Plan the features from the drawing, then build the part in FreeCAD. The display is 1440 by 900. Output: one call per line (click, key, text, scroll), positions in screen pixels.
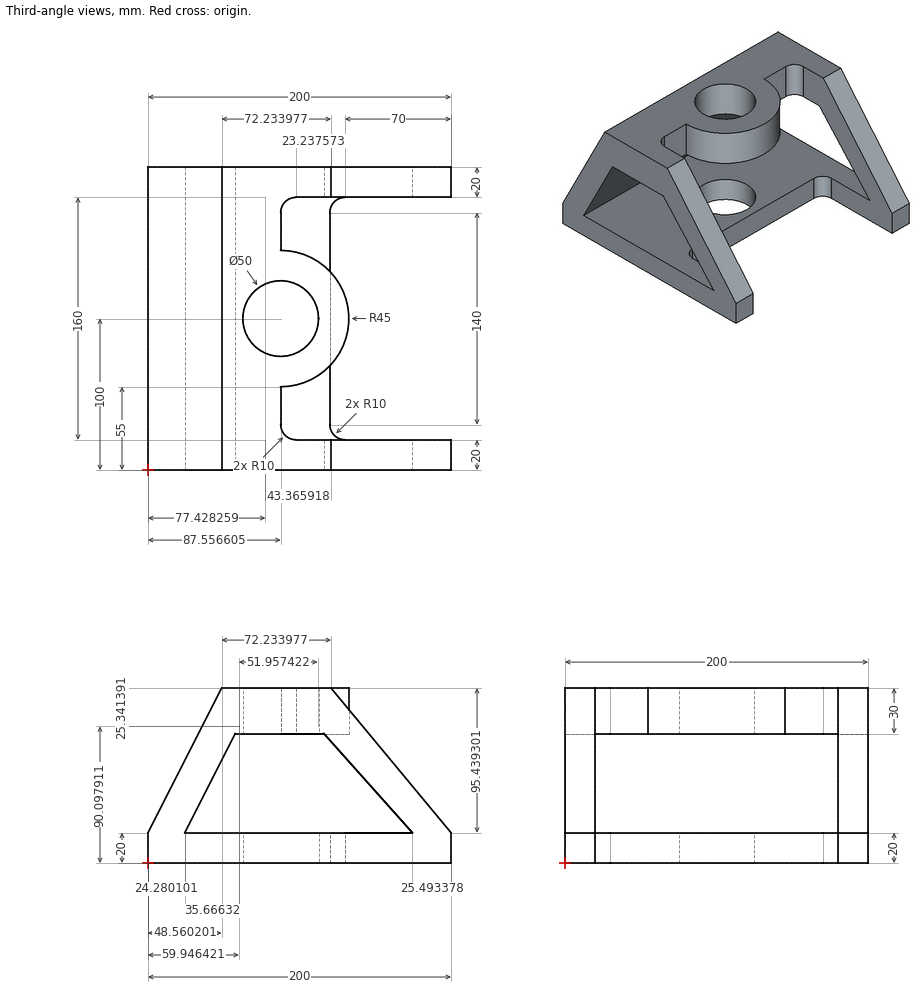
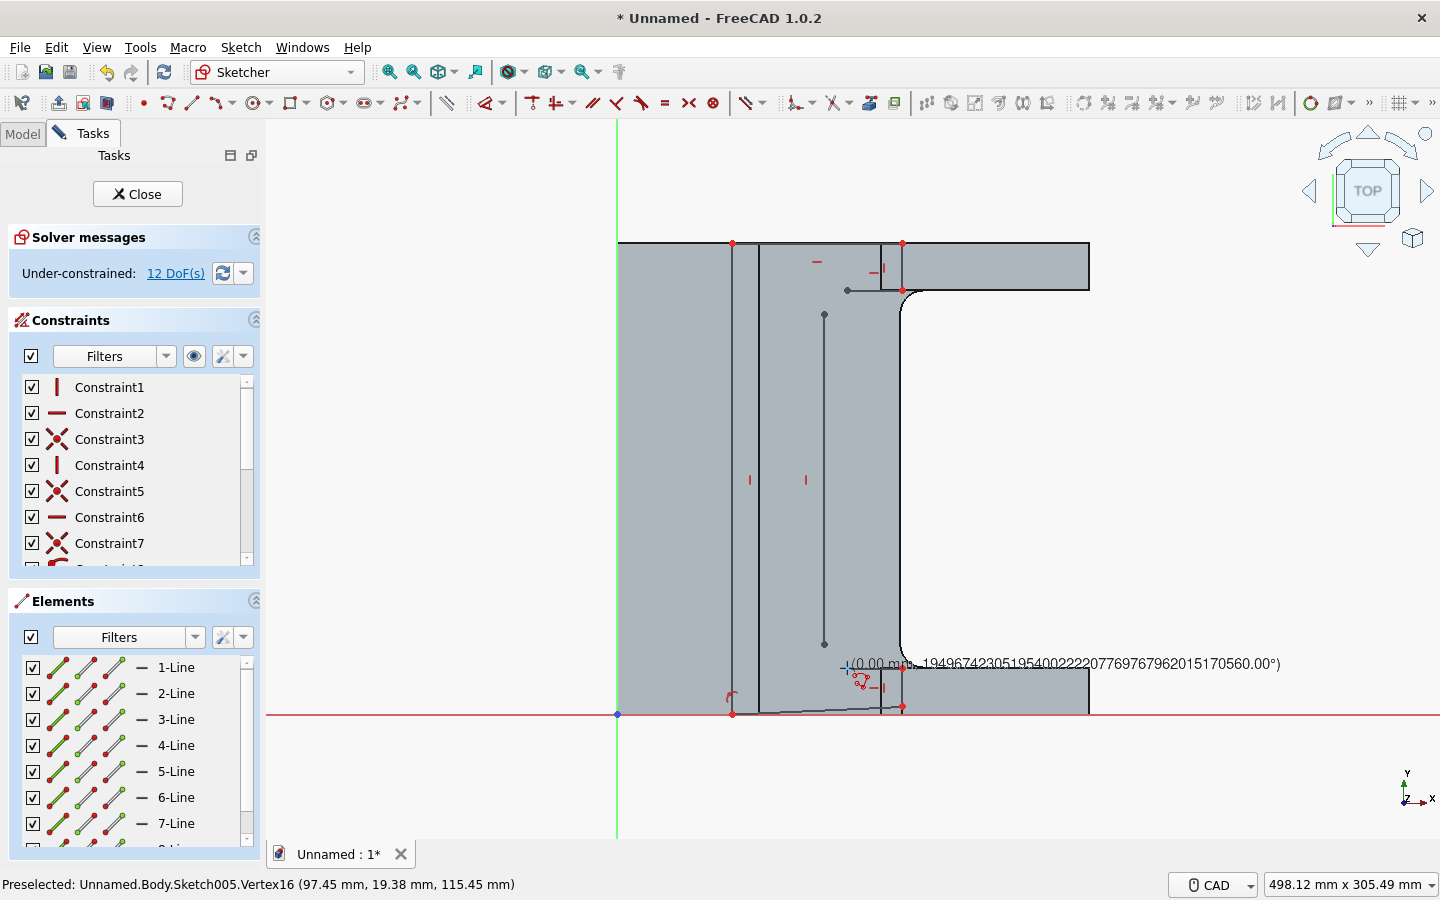
click(216, 104)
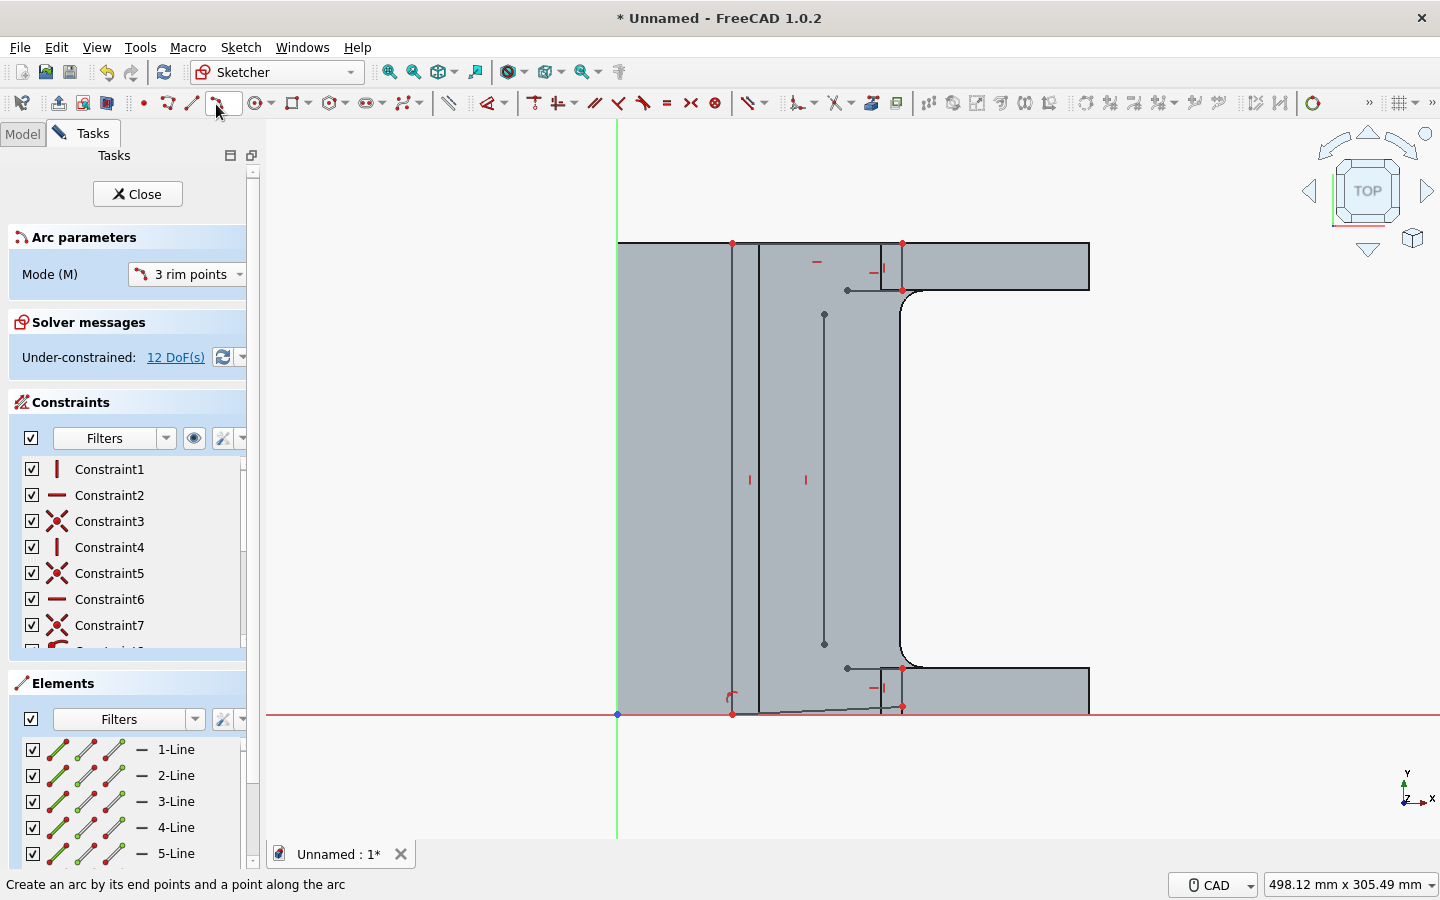
click(824, 315)
click(847, 291)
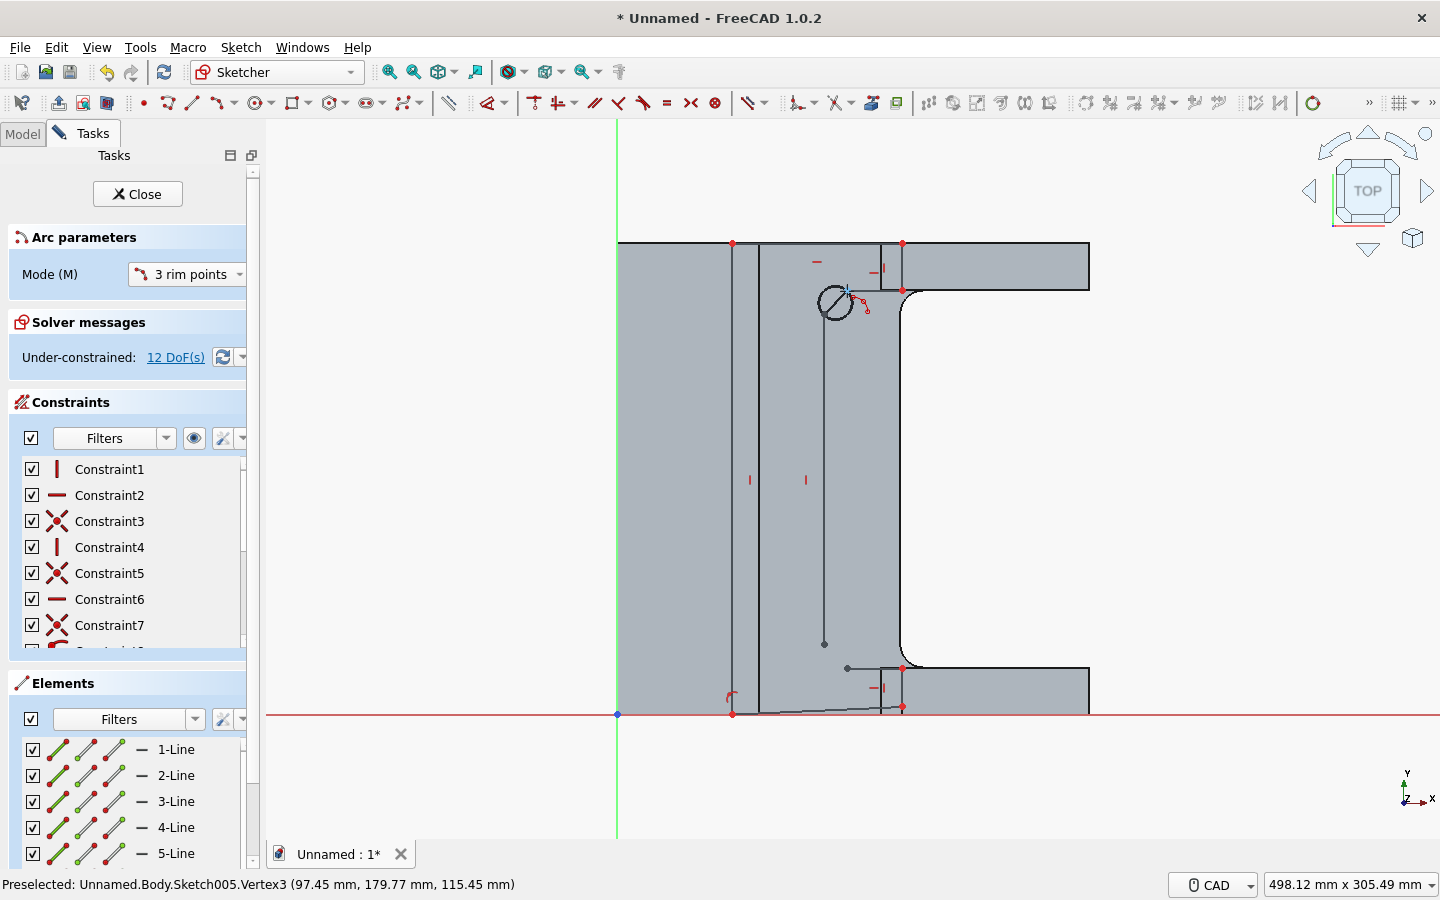
scroll(831, 297, up, 5)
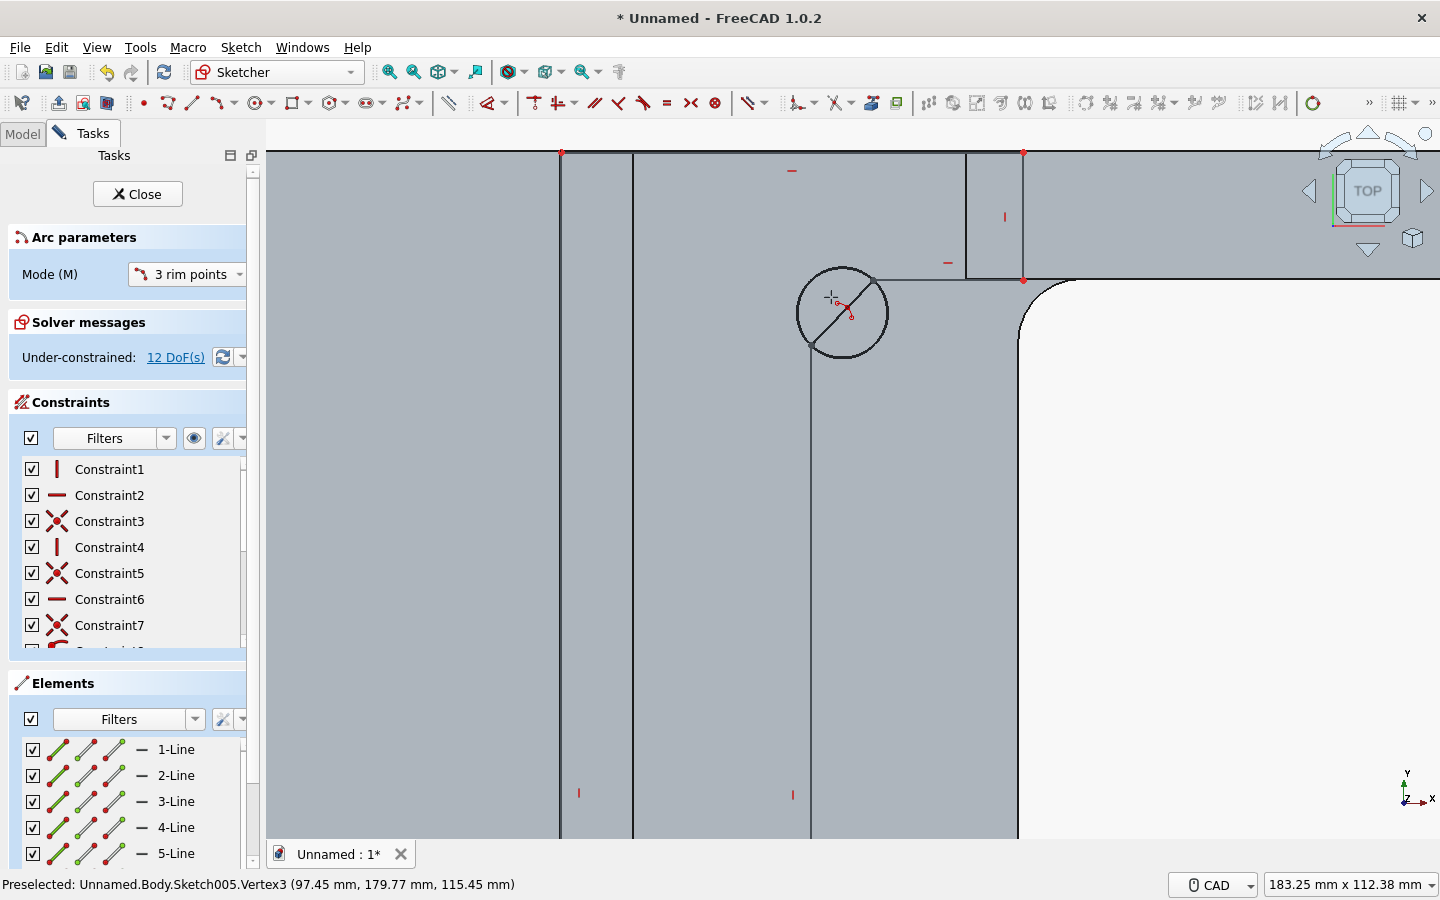
click(829, 298)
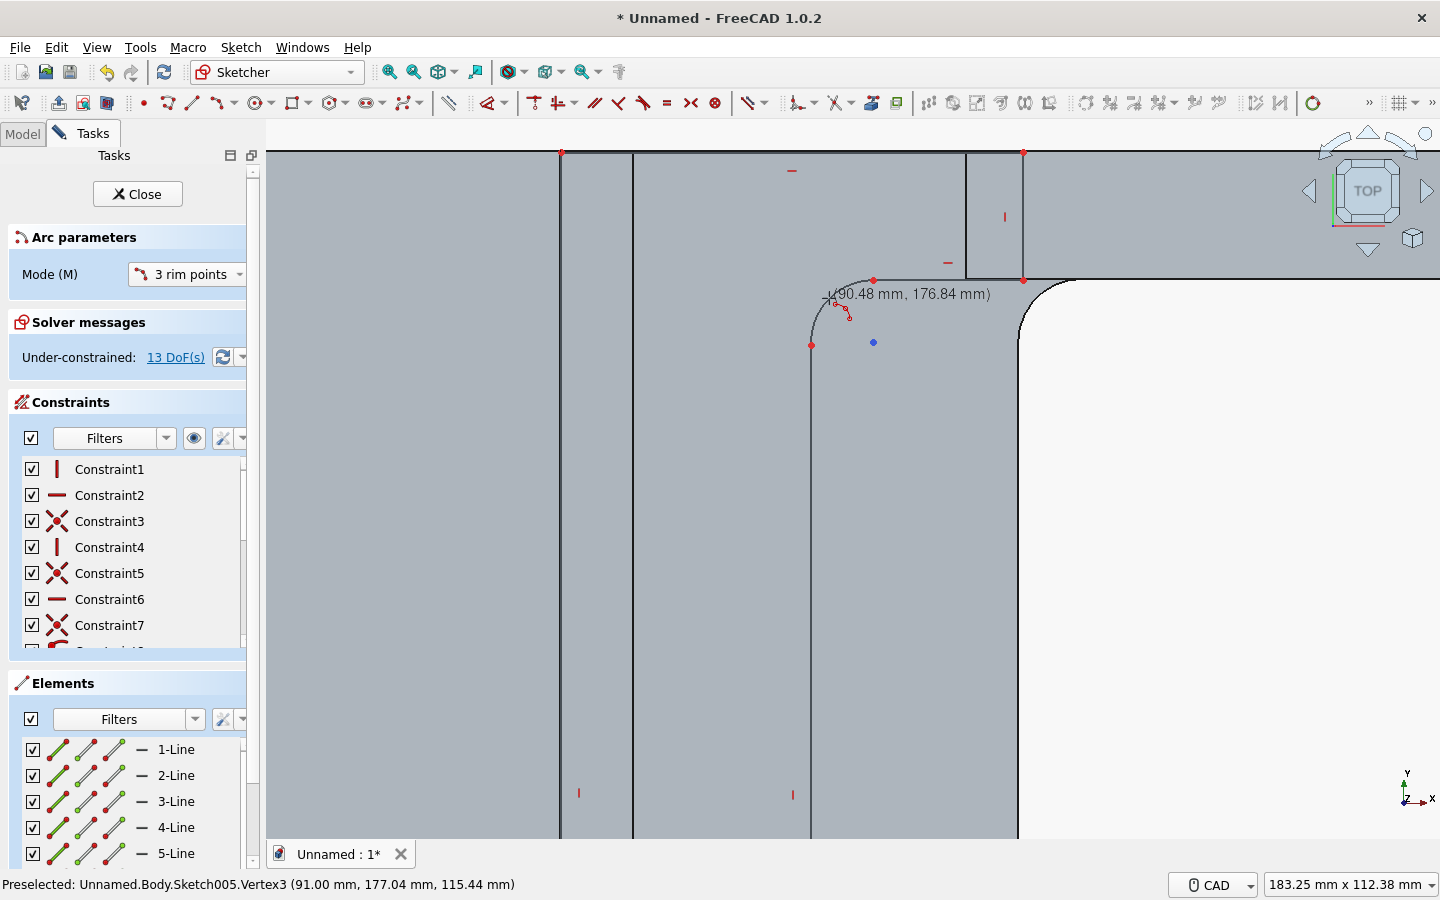
scroll(871, 297, down, 5)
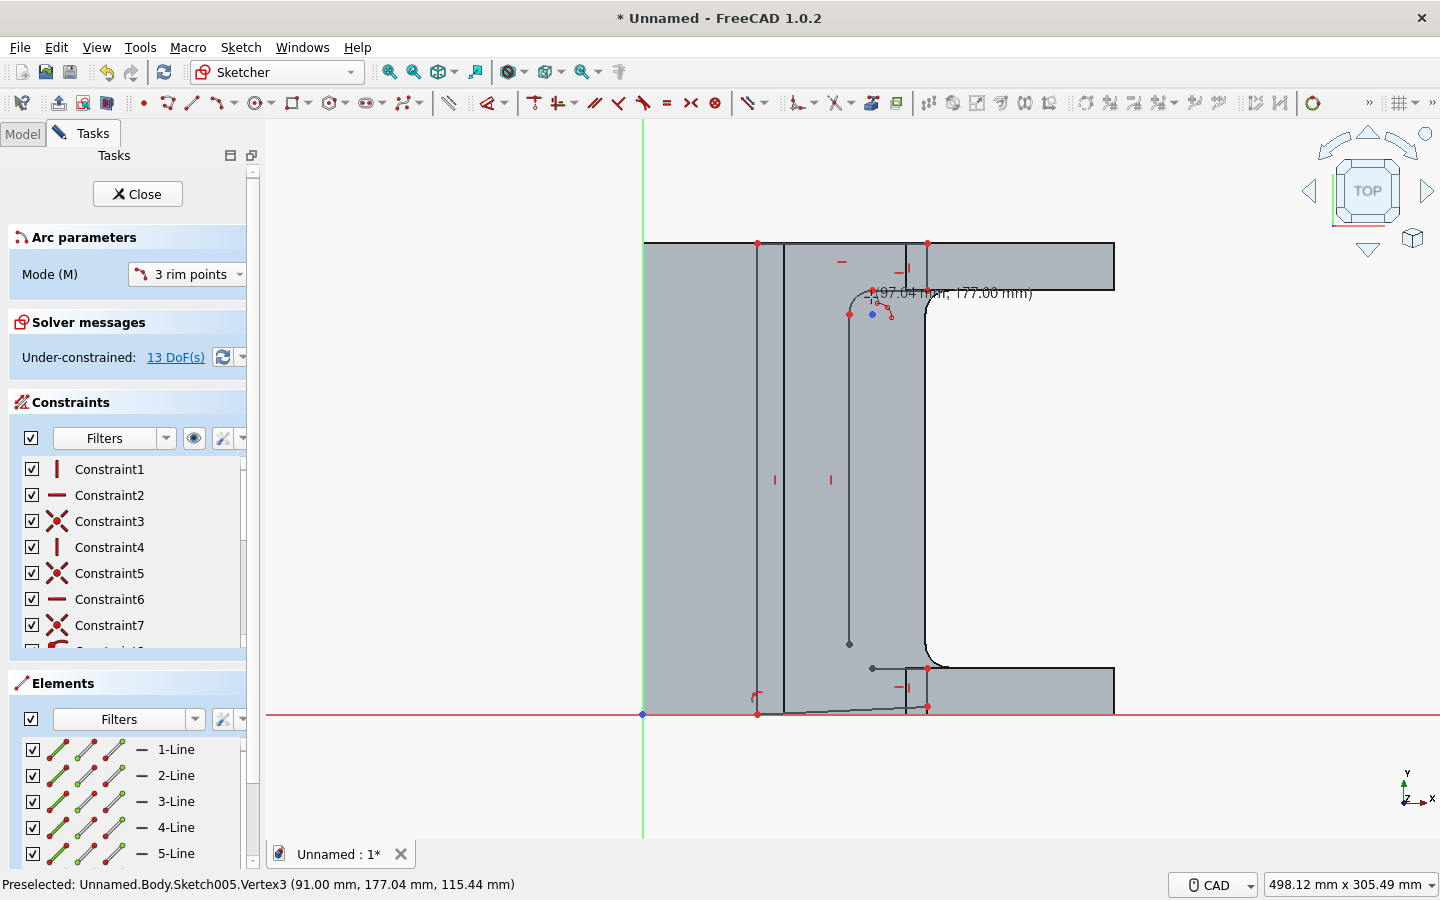
click(872, 669)
click(849, 645)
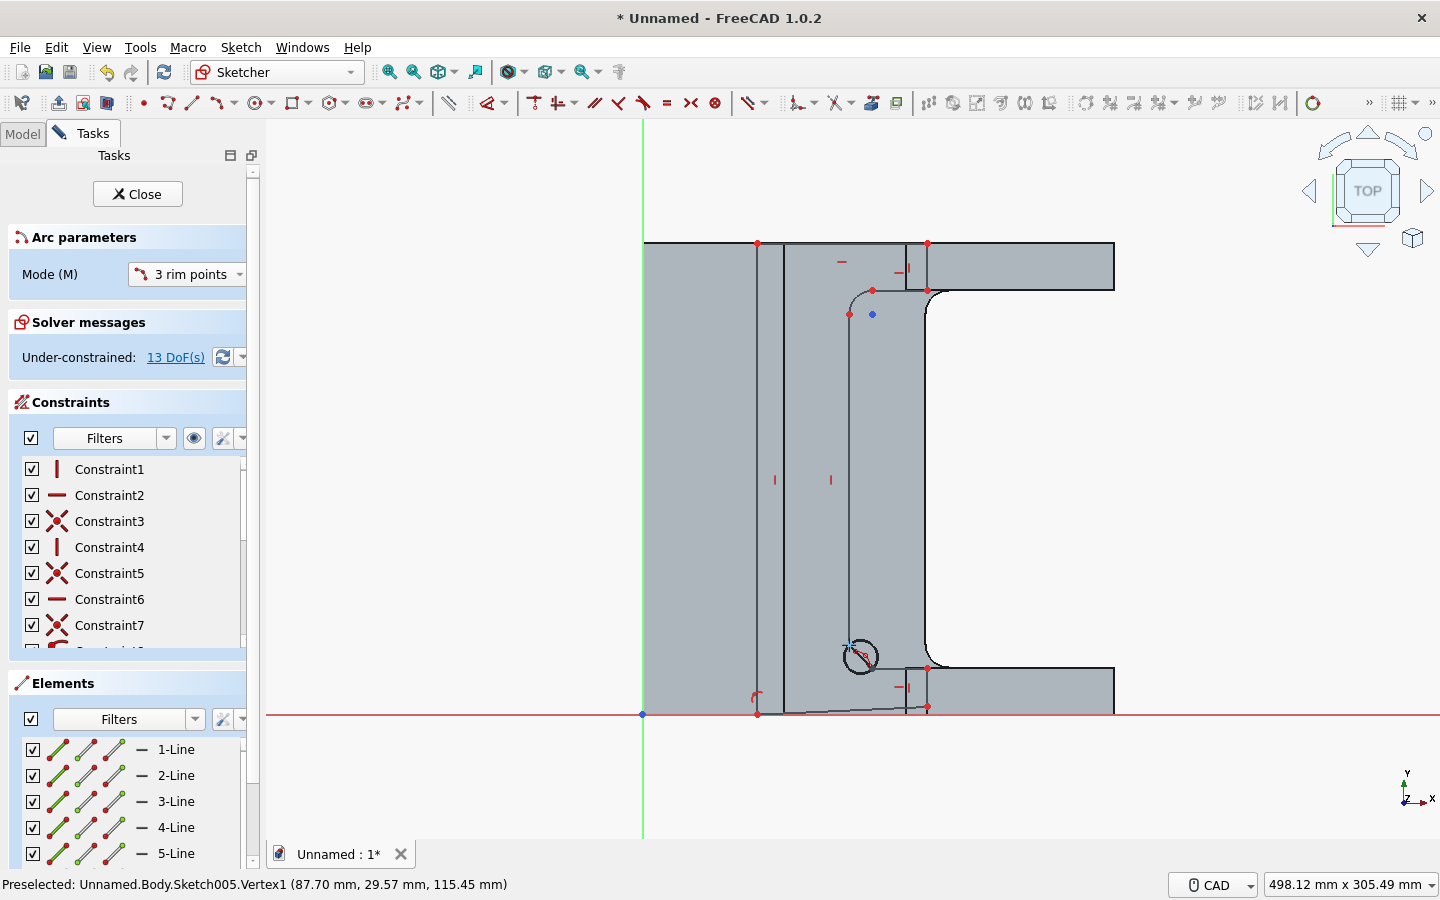
scroll(856, 661, up, 5)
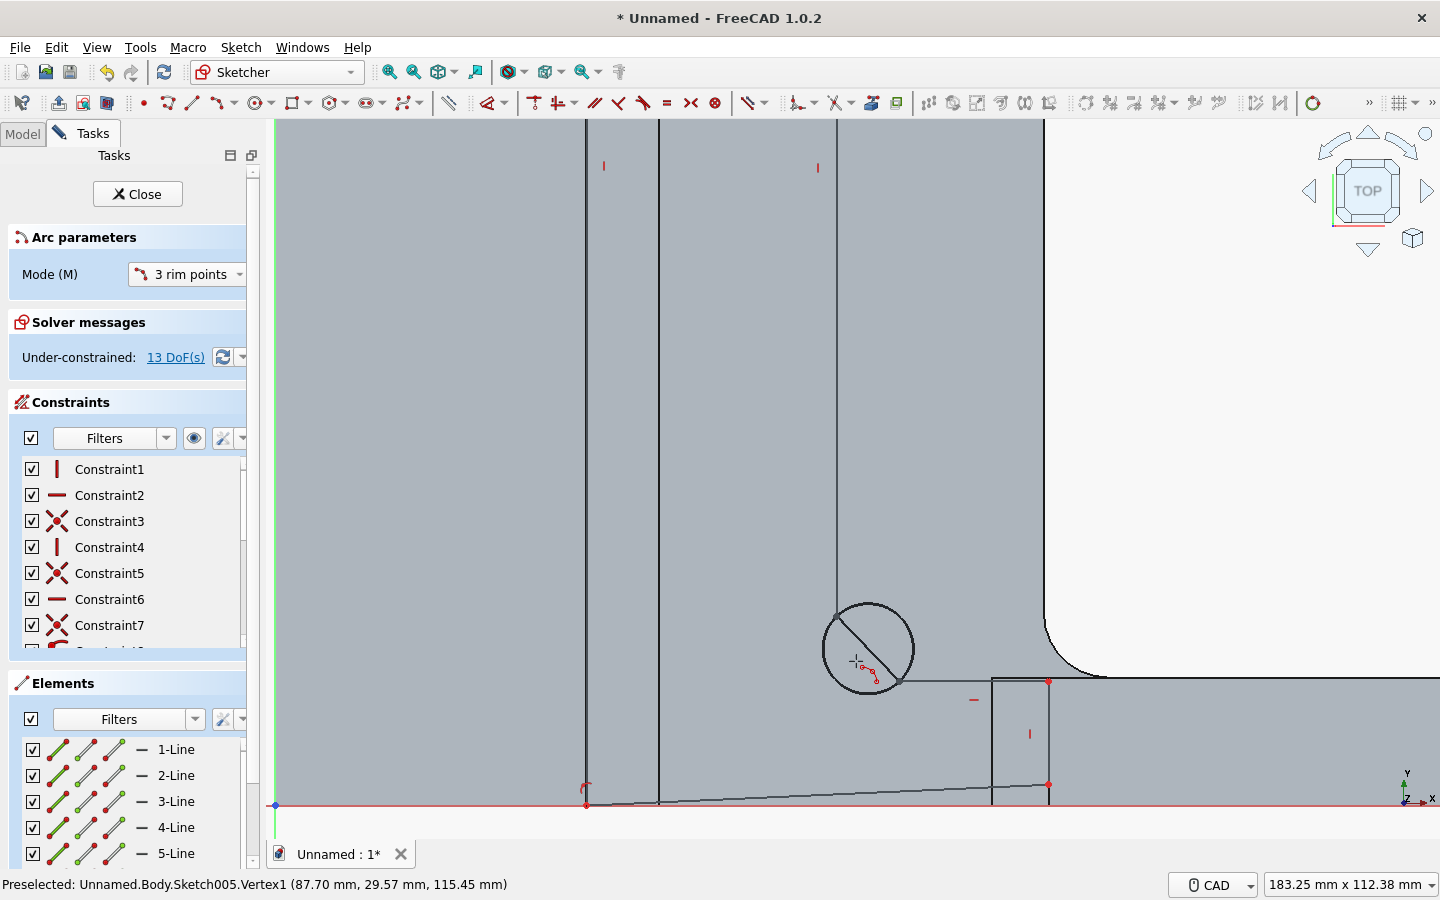
click(855, 659)
key(Escape)